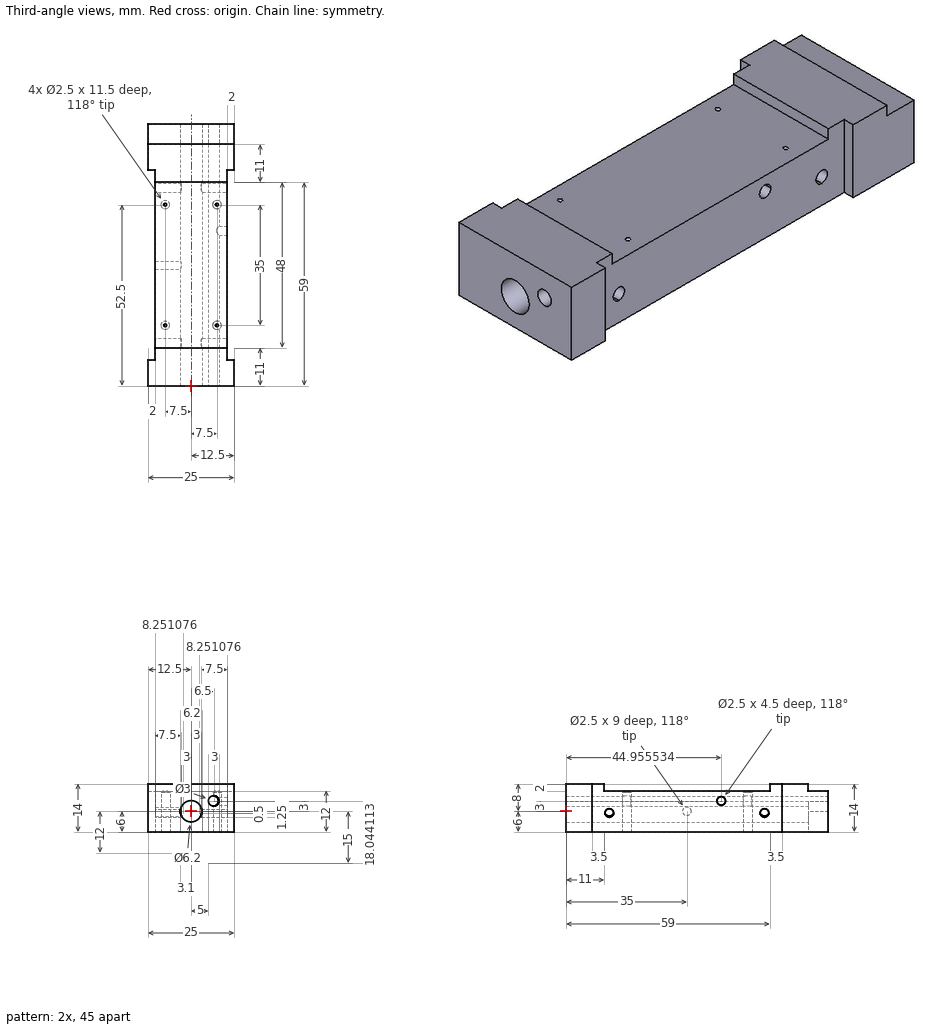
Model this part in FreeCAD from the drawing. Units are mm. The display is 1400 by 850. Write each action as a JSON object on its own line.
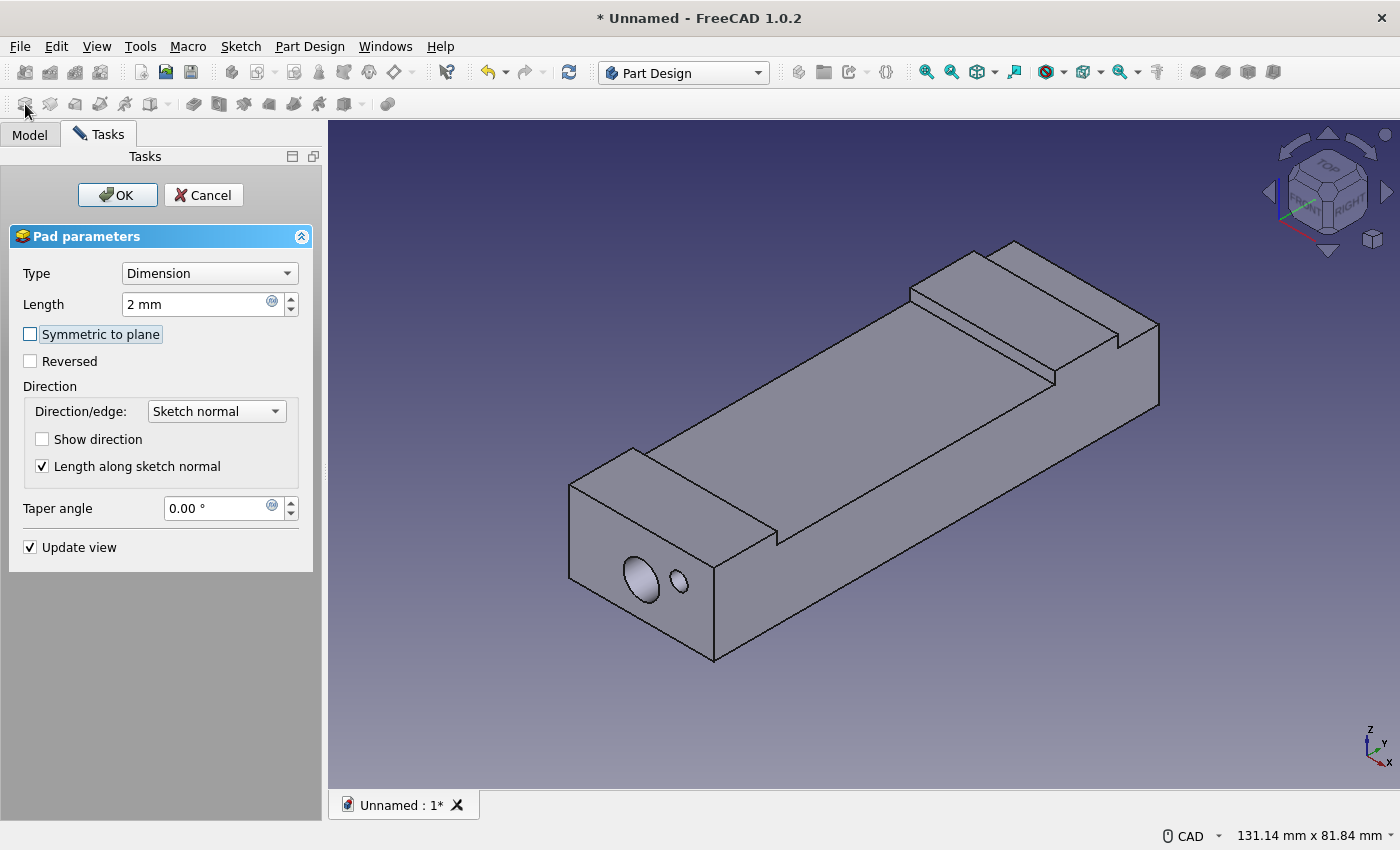
{"action": "left_click", "coordinate": [118, 195]}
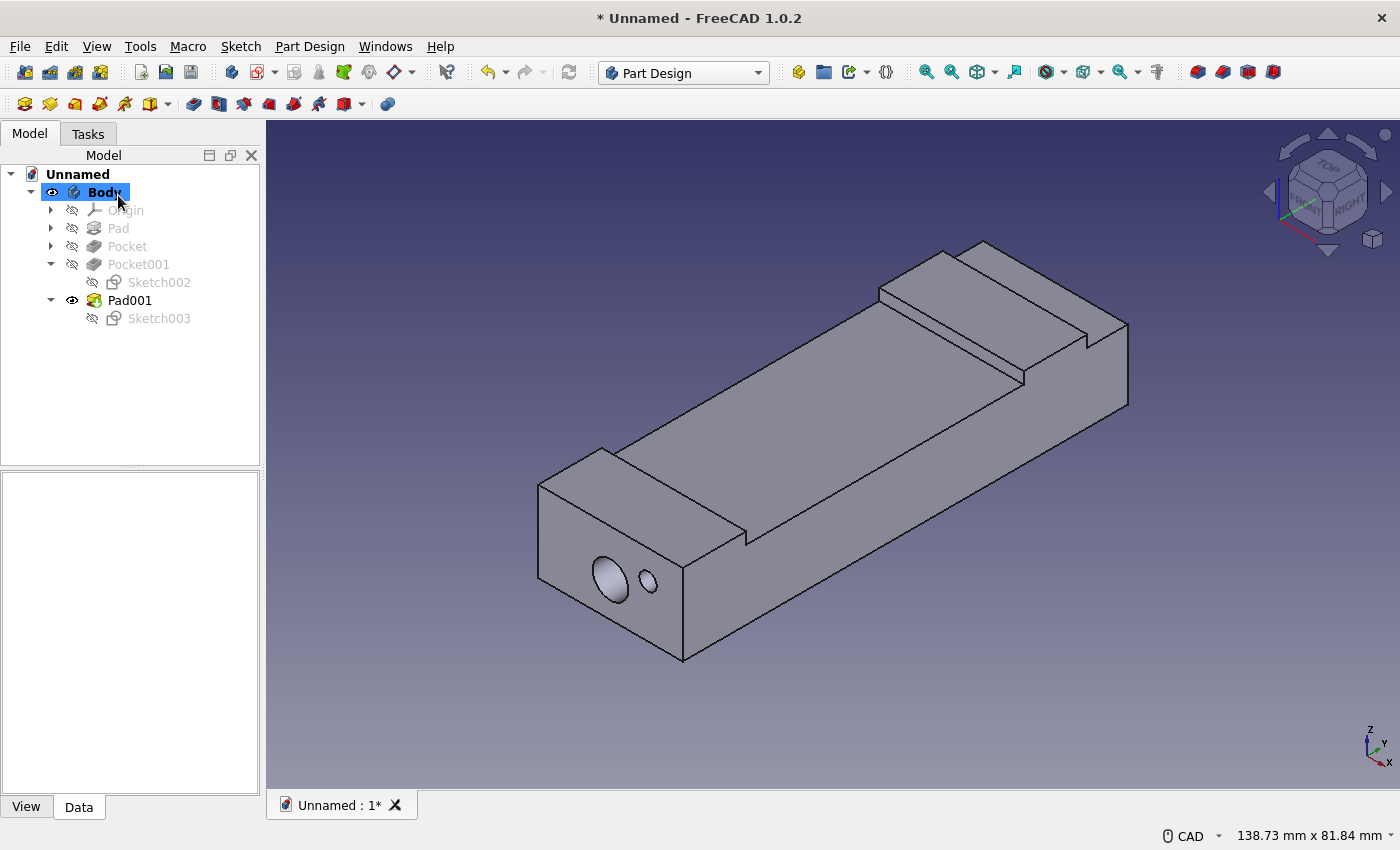
{"action": "left_click", "coordinate": [663, 519]}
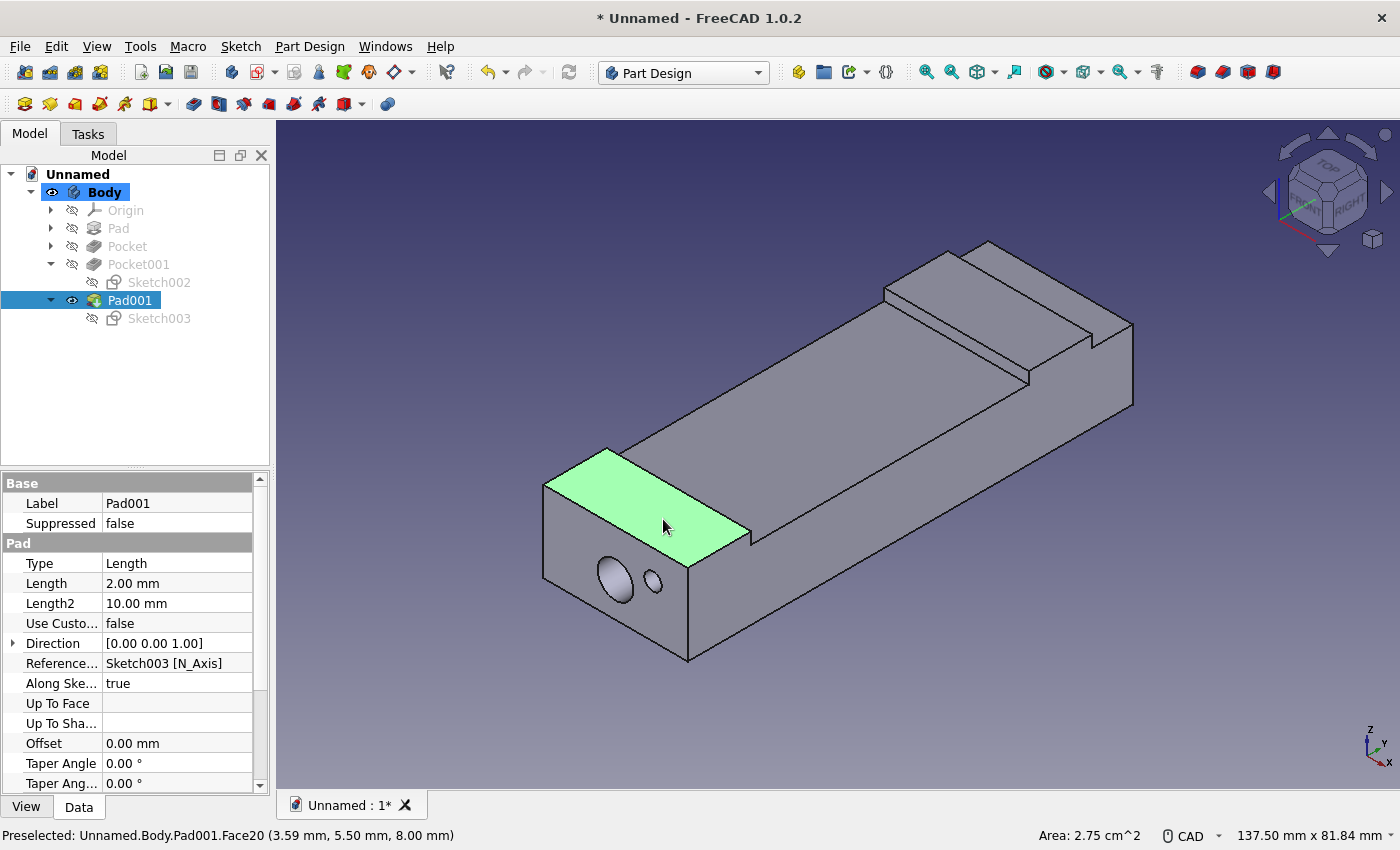
{"action": "left_click", "coordinate": [256, 72]}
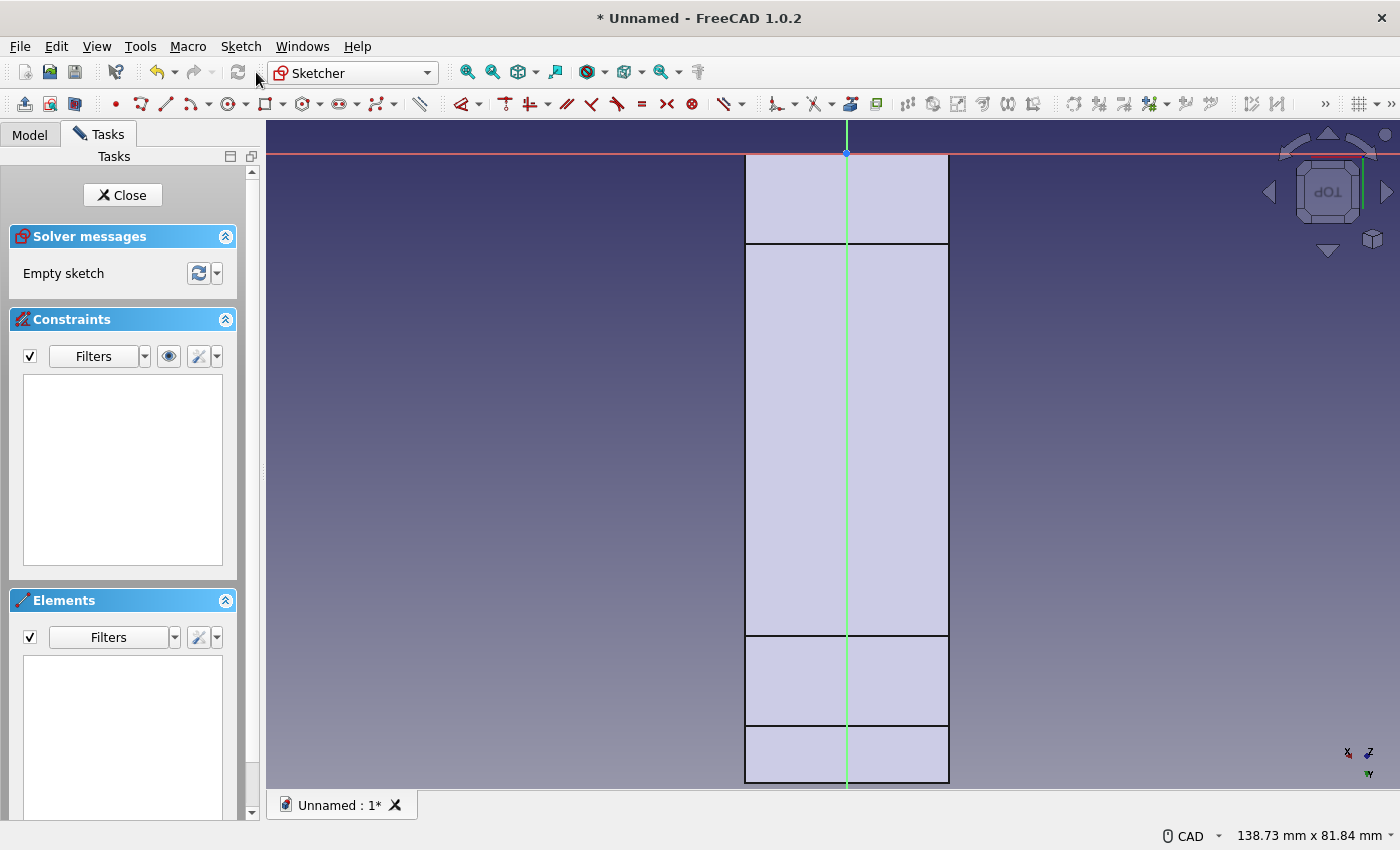
{"action": "scroll", "coordinate": [393, 724], "scroll_direction": "down", "scroll_amount": 1}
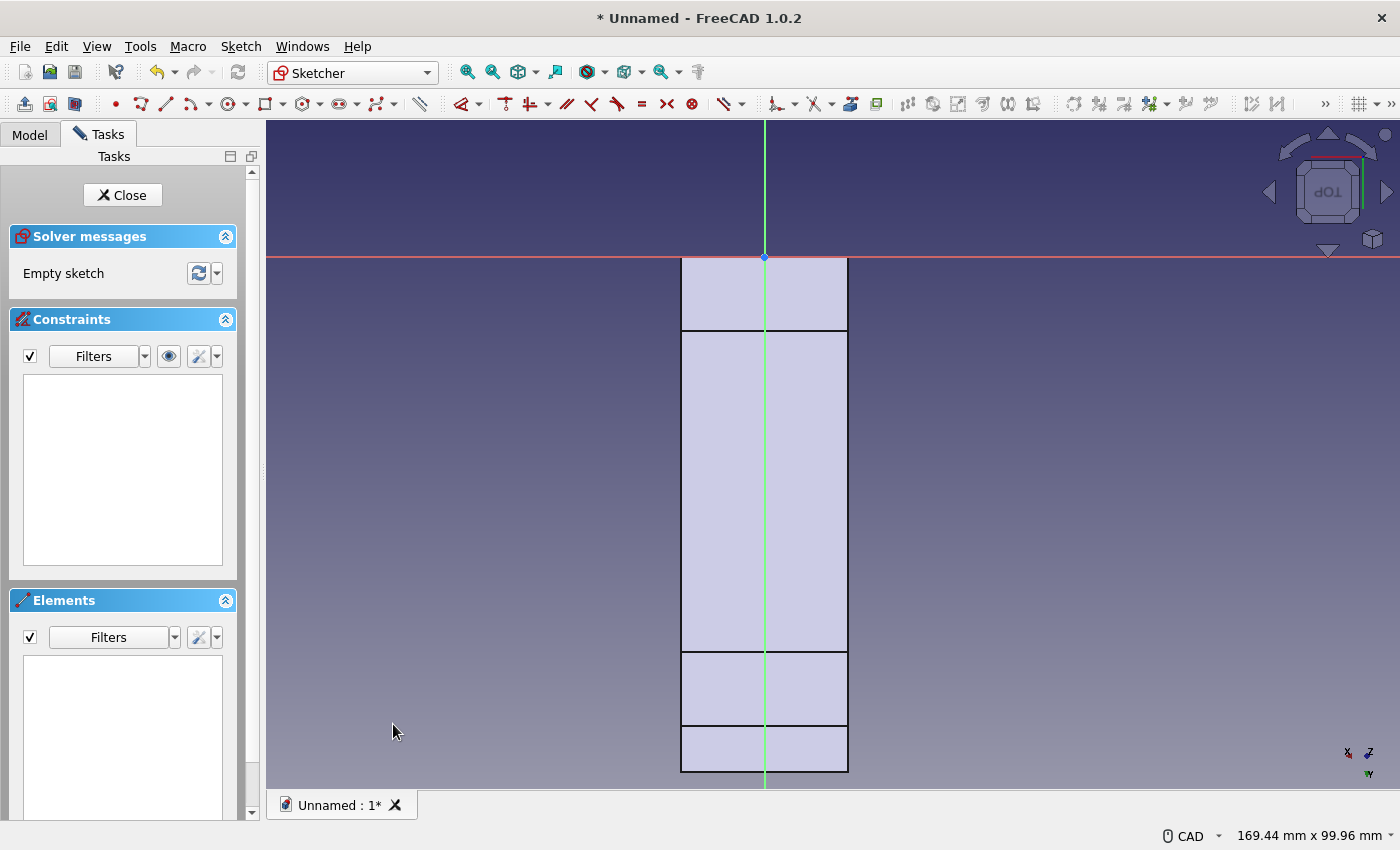
{"action": "left_click", "coordinate": [264, 104]}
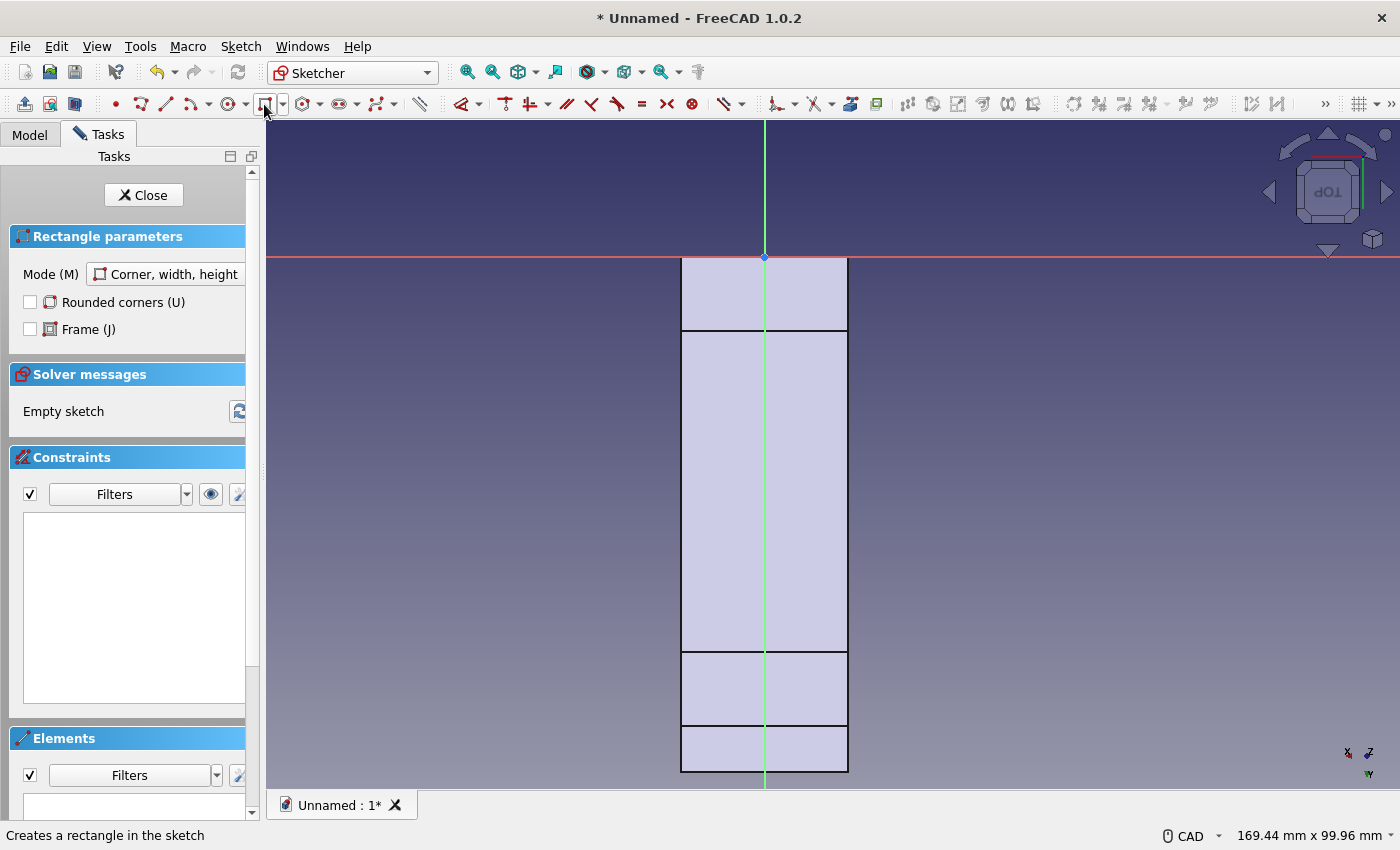
{"action": "left_click", "coordinate": [681, 331]}
{"action": "left_click", "coordinate": [694, 652]}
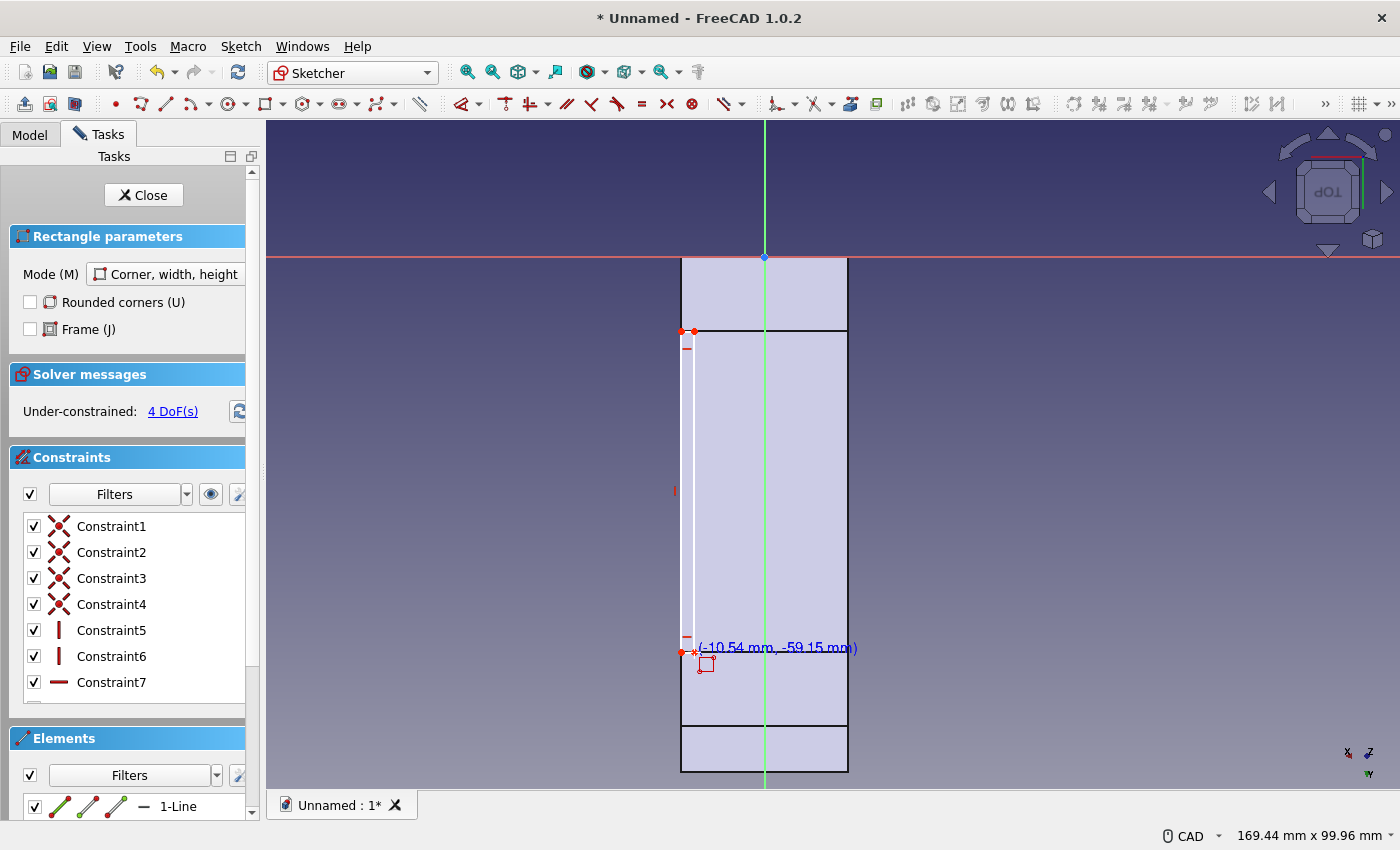
{"action": "left_click", "coordinate": [835, 331]}
{"action": "left_click", "coordinate": [848, 652]}
{"action": "key", "text": "Escape"}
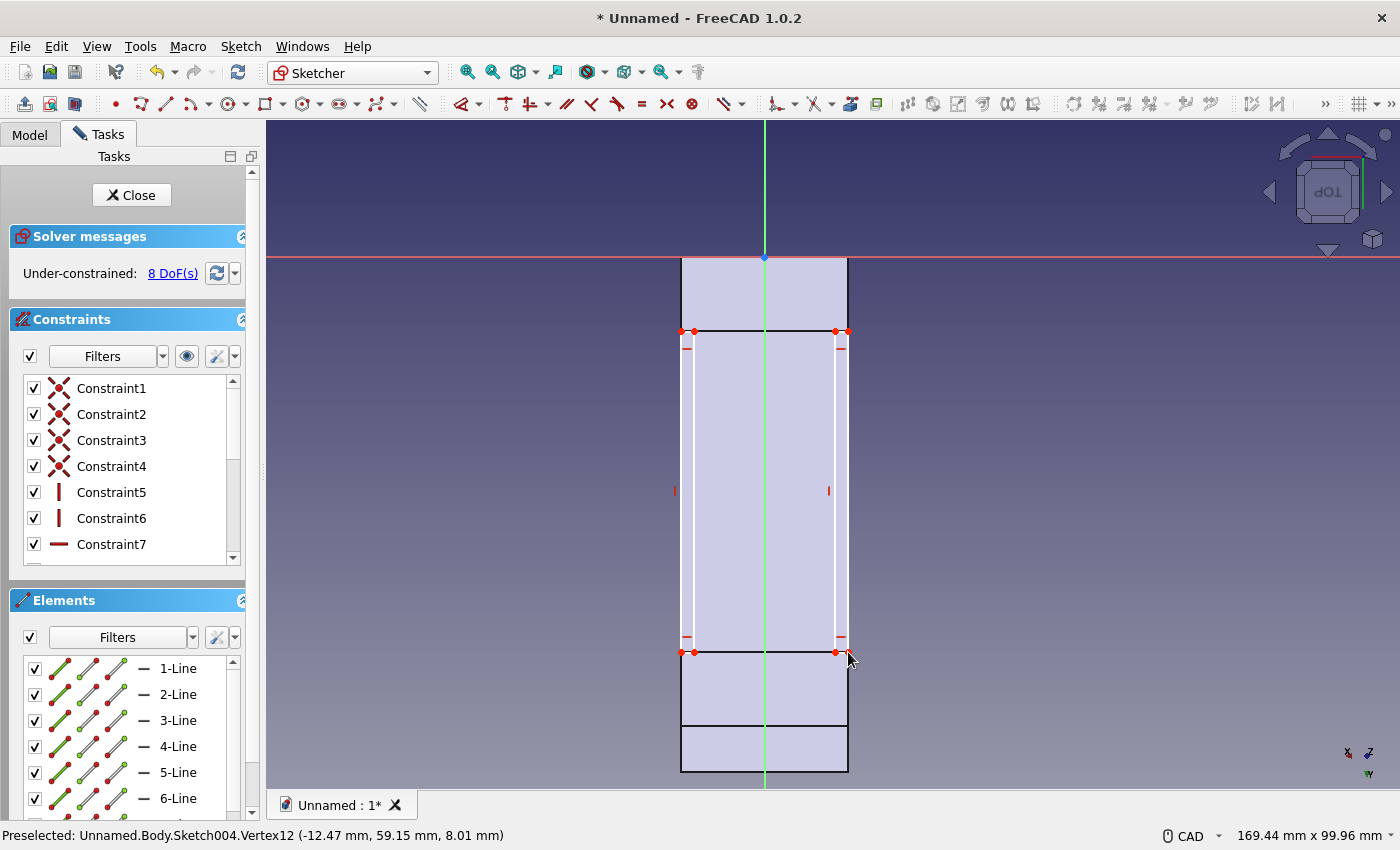
{"action": "left_click", "coordinate": [694, 332]}